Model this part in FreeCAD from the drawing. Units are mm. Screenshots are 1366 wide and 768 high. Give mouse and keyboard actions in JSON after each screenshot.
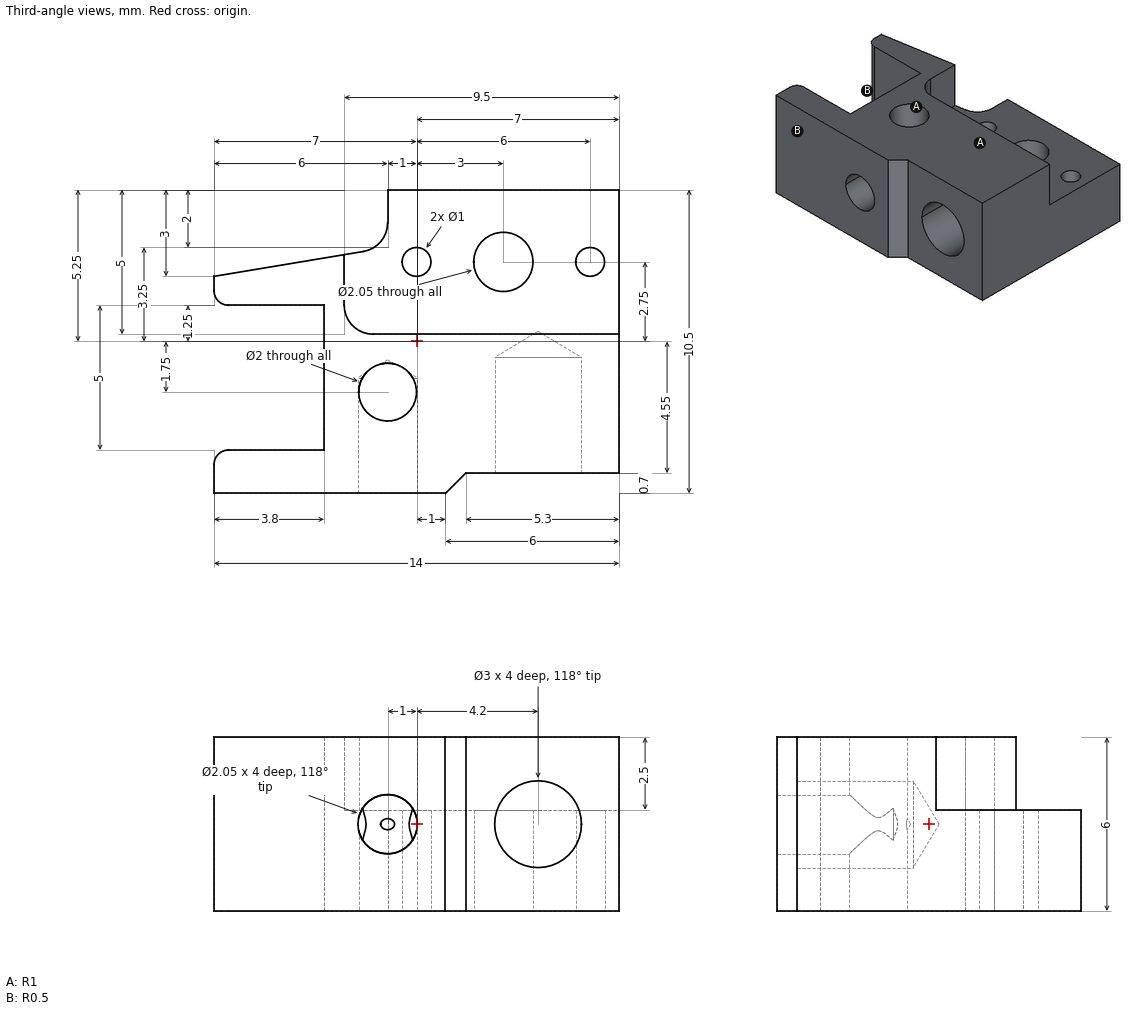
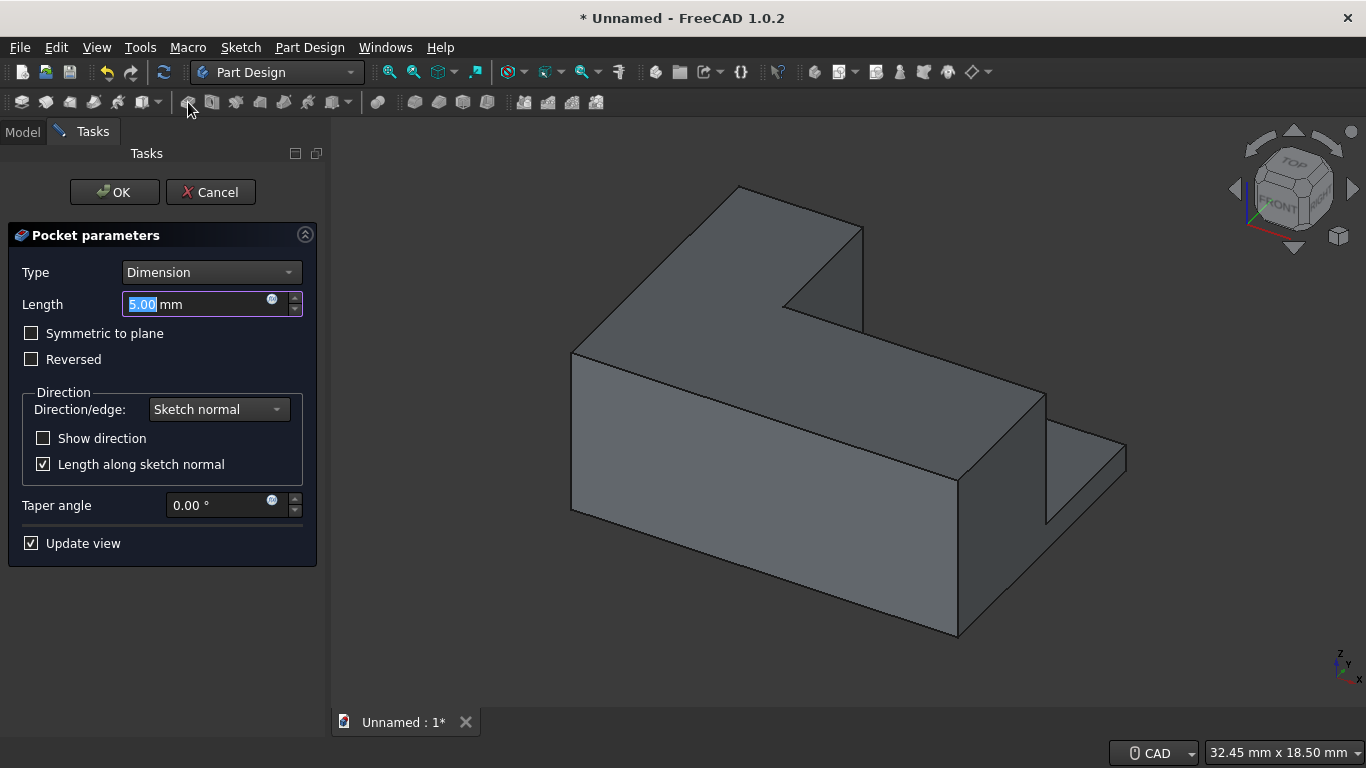
{"action": "type", "text": "2.5"}
{"action": "key", "text": "Tab"}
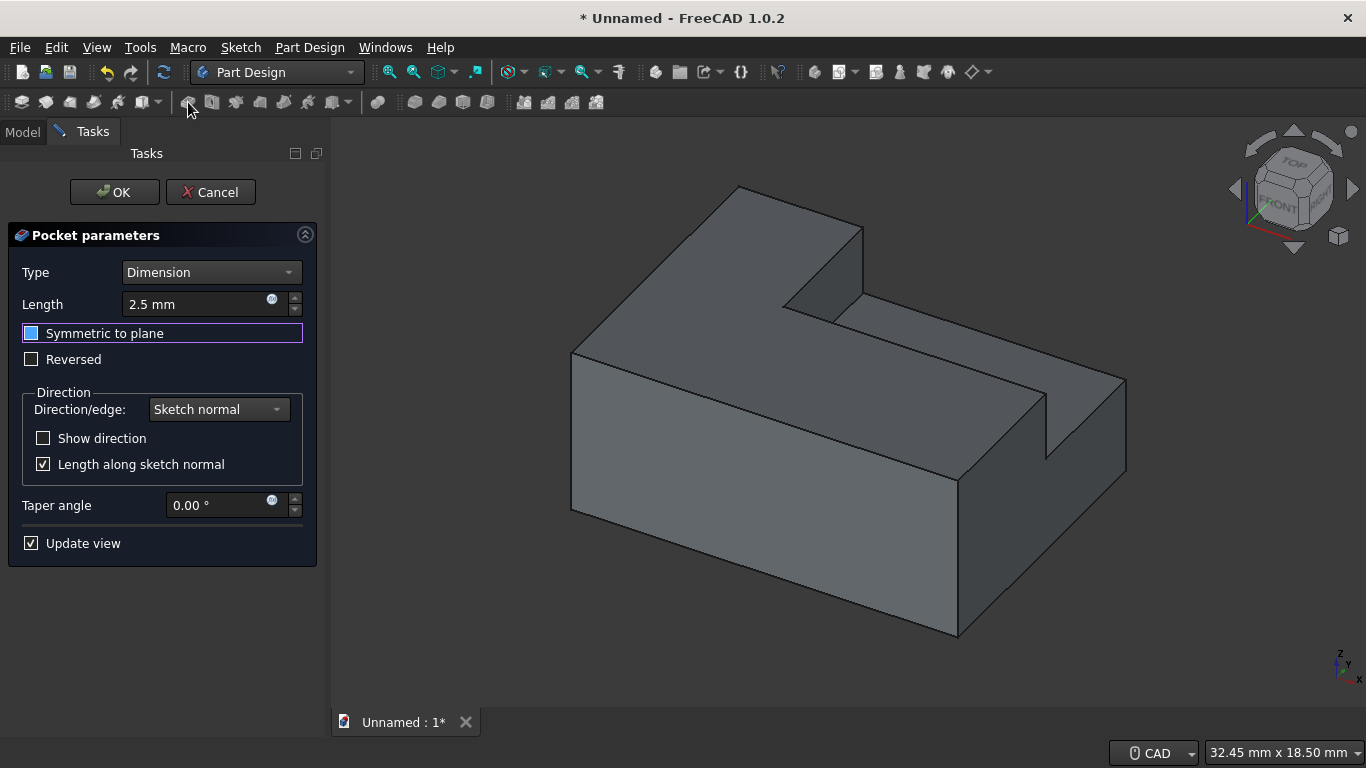
{"action": "left_click", "coordinate": [115, 192]}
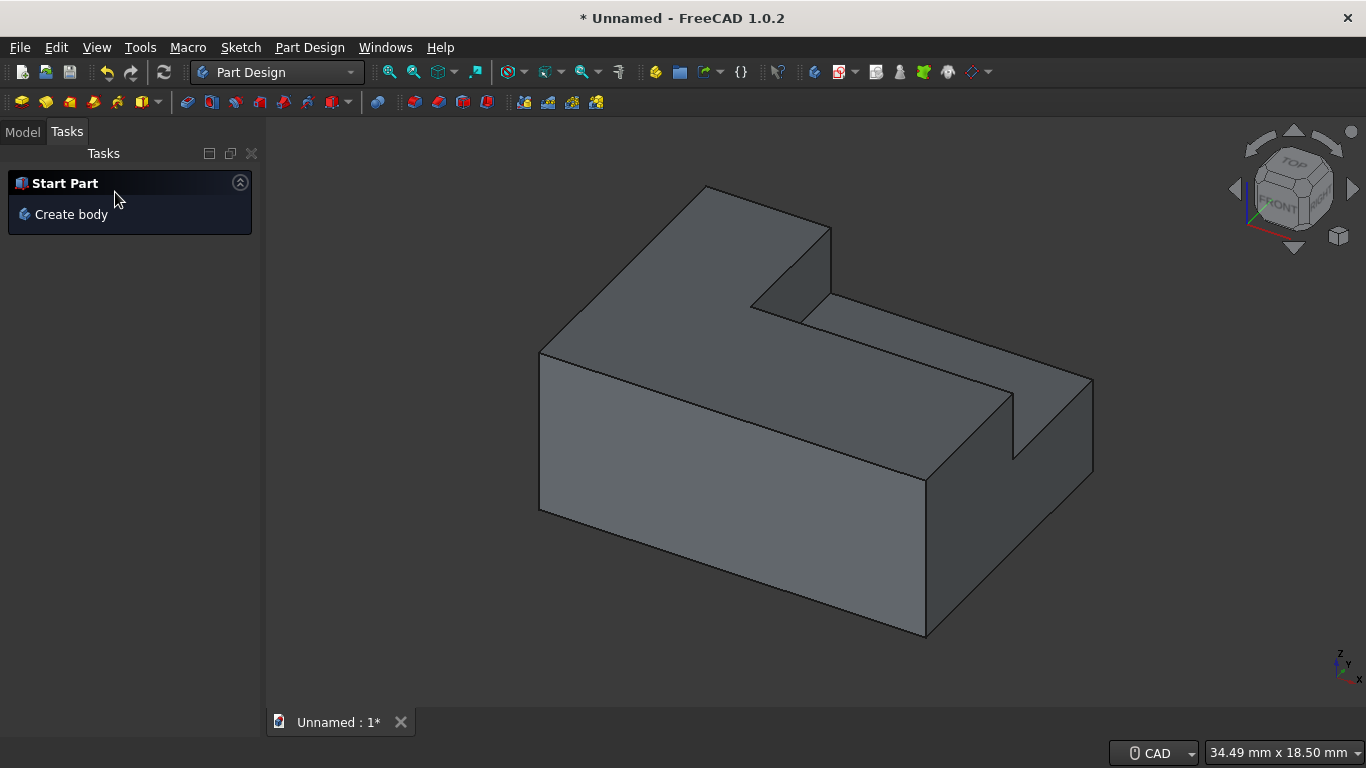
{"action": "left_click", "coordinate": [682, 320]}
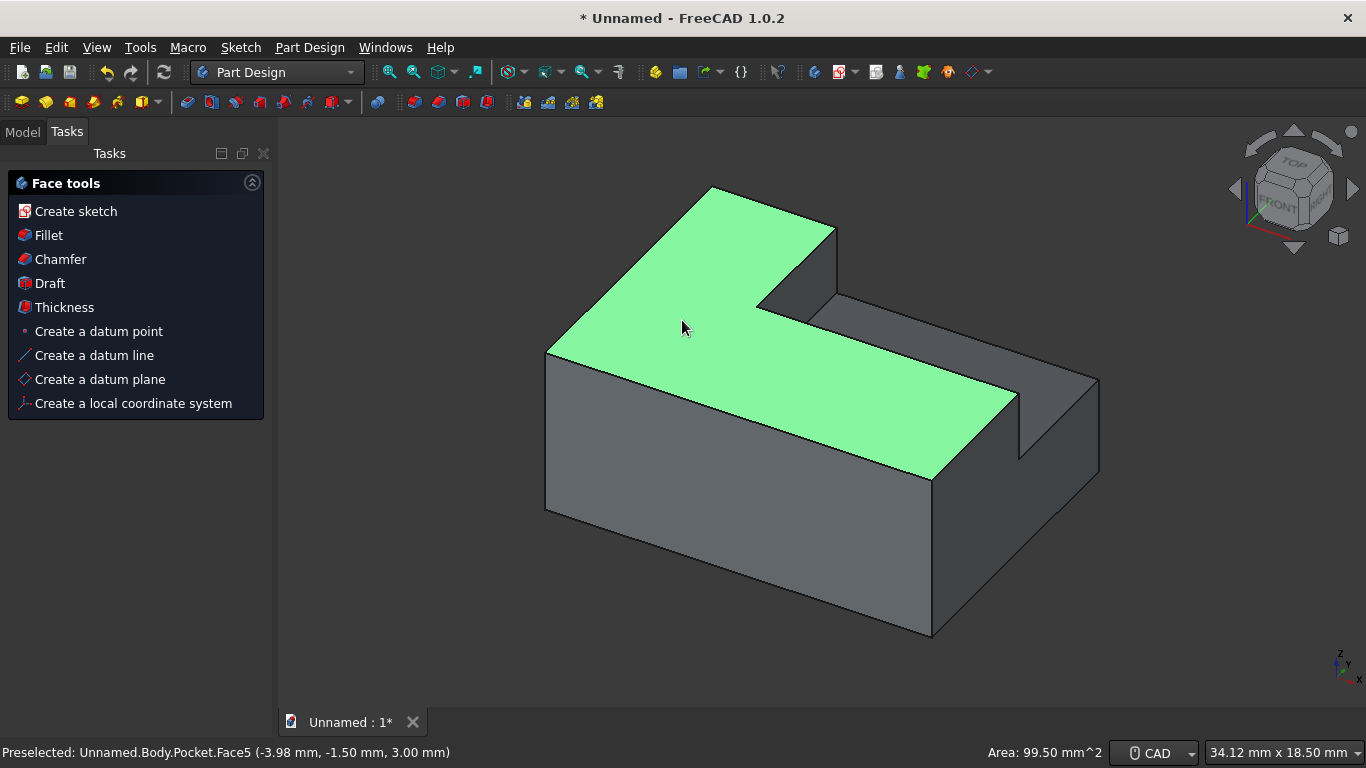
{"action": "left_click", "coordinate": [840, 72]}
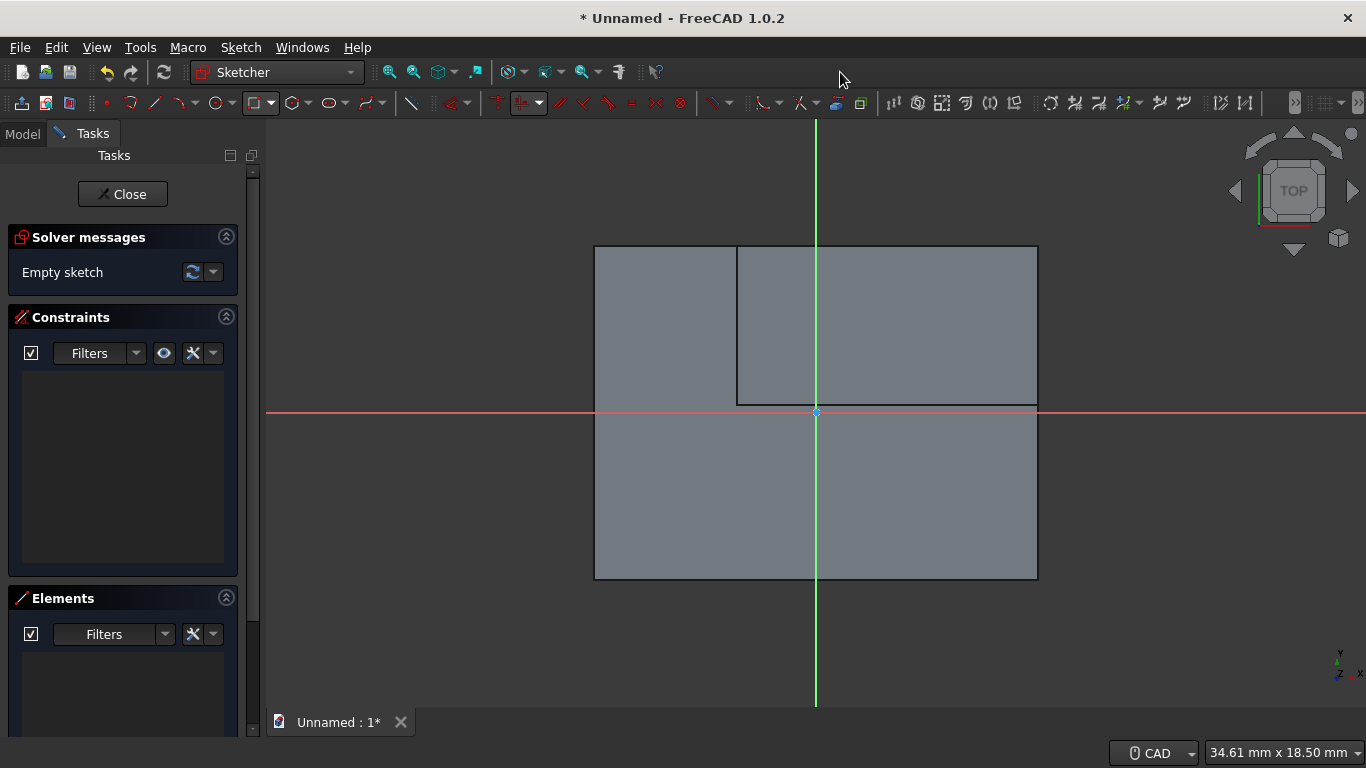
{"action": "scroll", "coordinate": [670, 261], "scroll_direction": "up", "scroll_amount": 4}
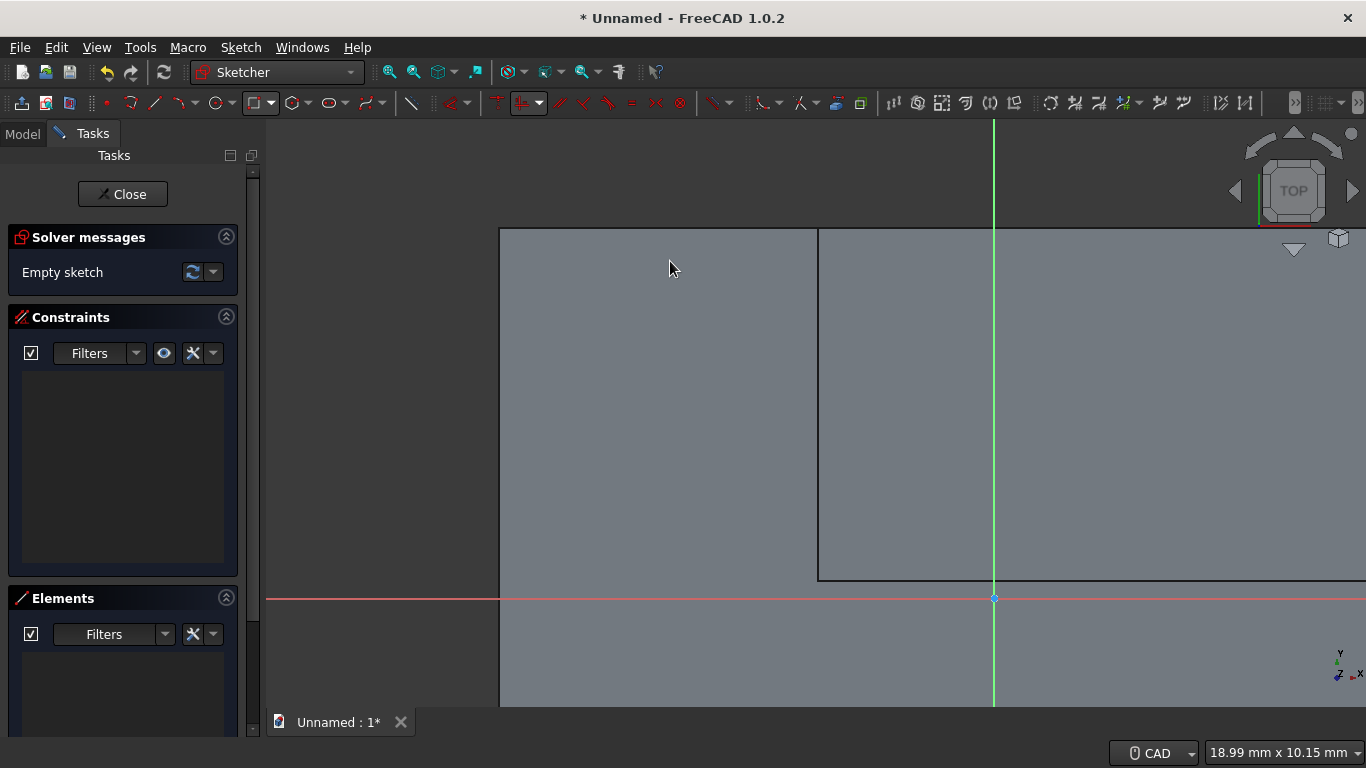
{"action": "left_click", "coordinate": [132, 104]}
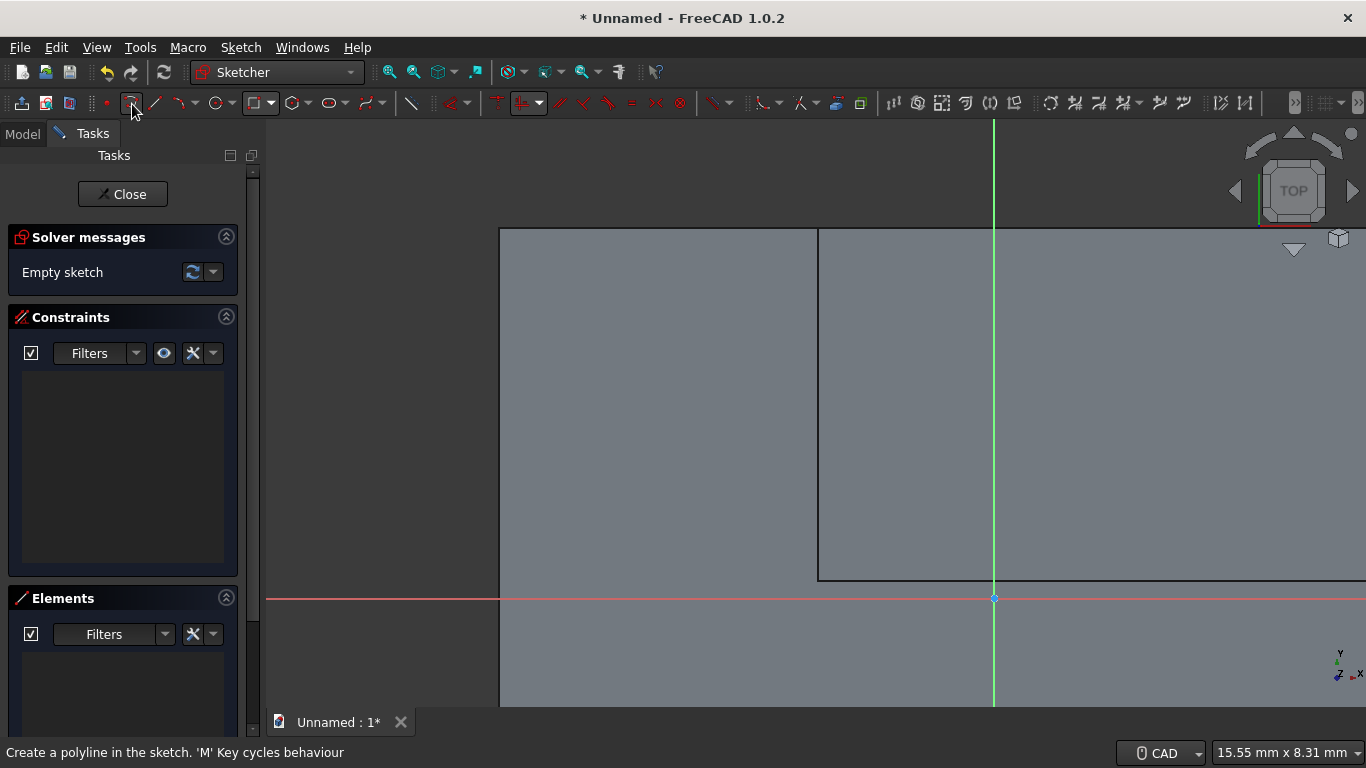
{"action": "left_click", "coordinate": [924, 369]}
{"action": "left_click", "coordinate": [924, 228]}
{"action": "left_click", "coordinate": [499, 228]}
{"action": "left_click", "coordinate": [499, 440]}
{"action": "left_click", "coordinate": [924, 370]}
{"action": "key", "text": "Escape"}
{"action": "key", "text": "Escape"}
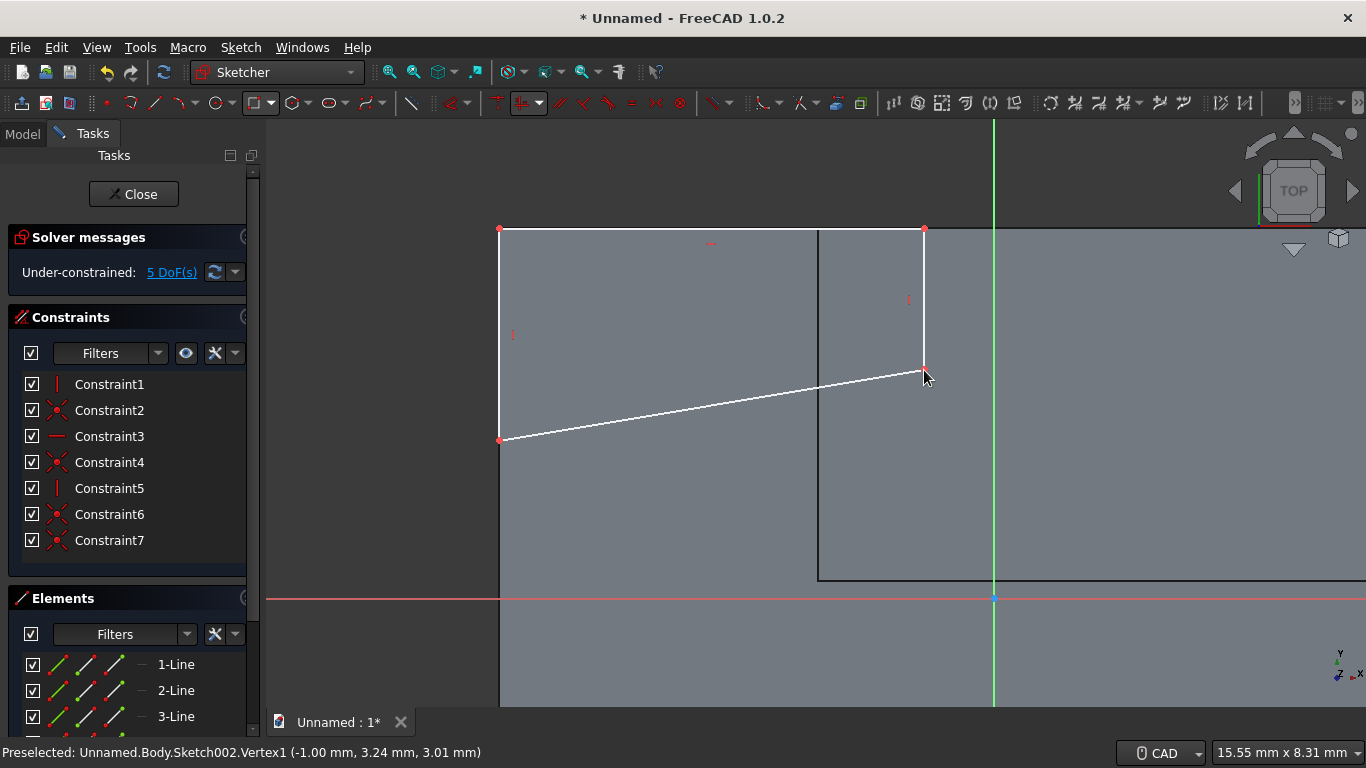
{"action": "left_click", "coordinate": [450, 104]}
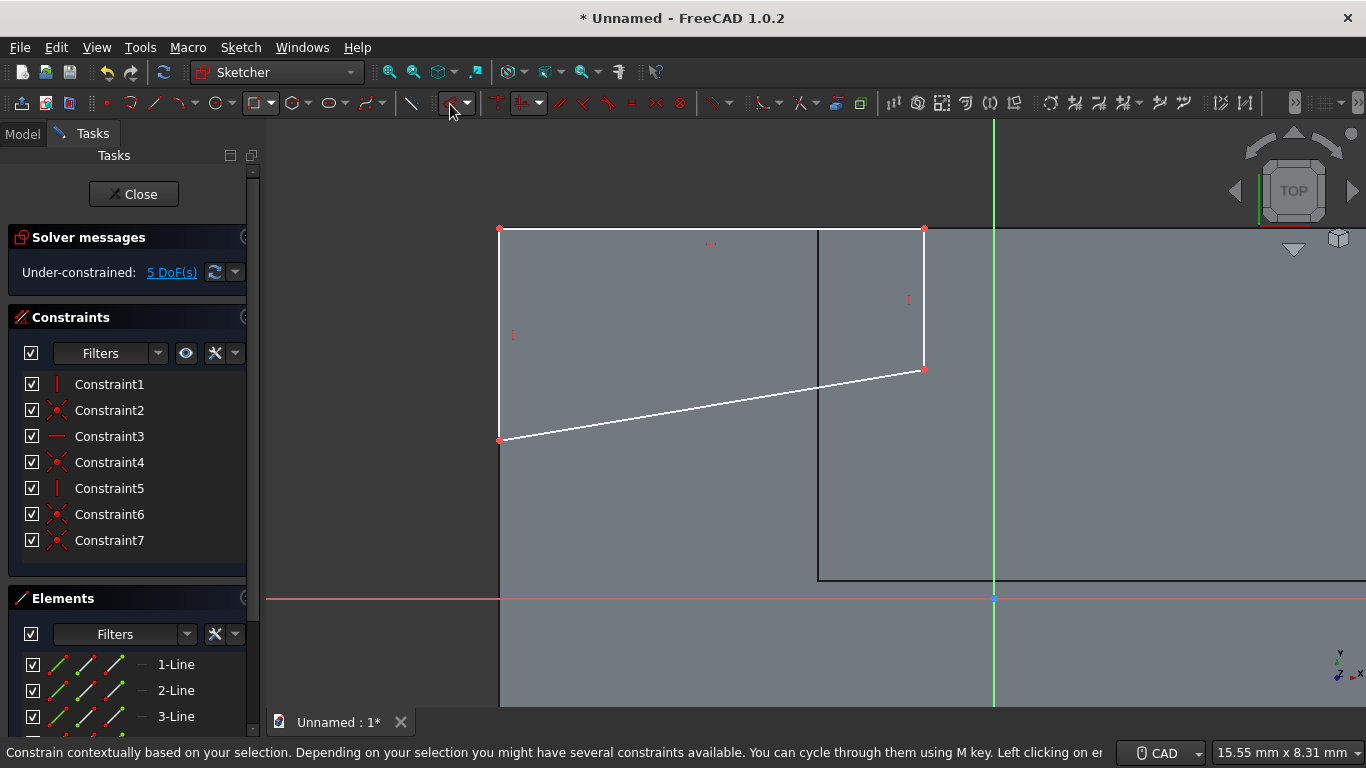
{"action": "left_click", "coordinate": [924, 328]}
{"action": "left_click", "coordinate": [958, 300]}